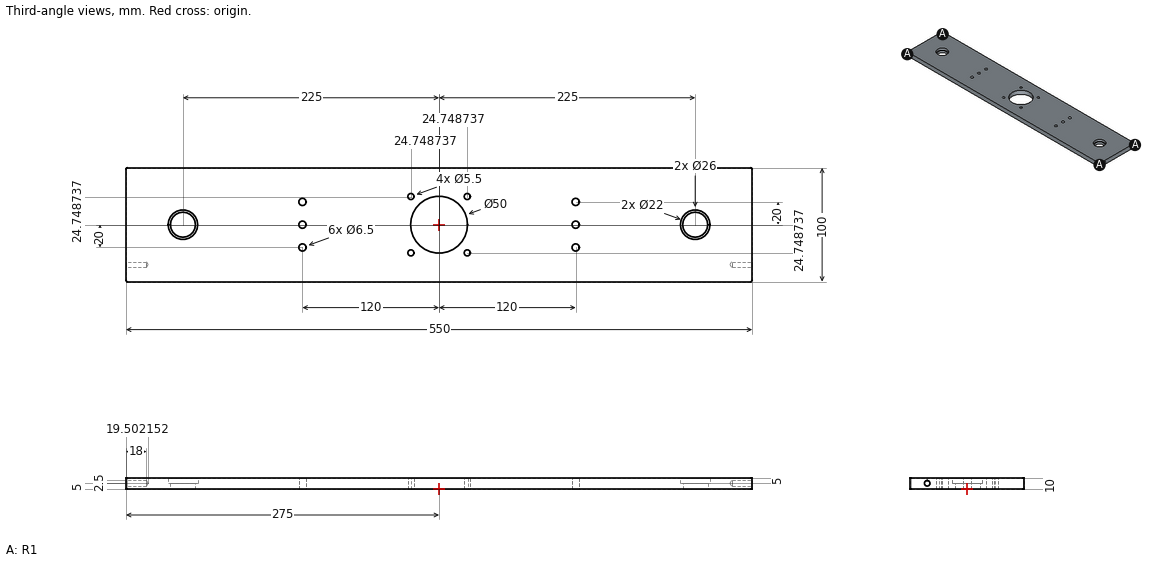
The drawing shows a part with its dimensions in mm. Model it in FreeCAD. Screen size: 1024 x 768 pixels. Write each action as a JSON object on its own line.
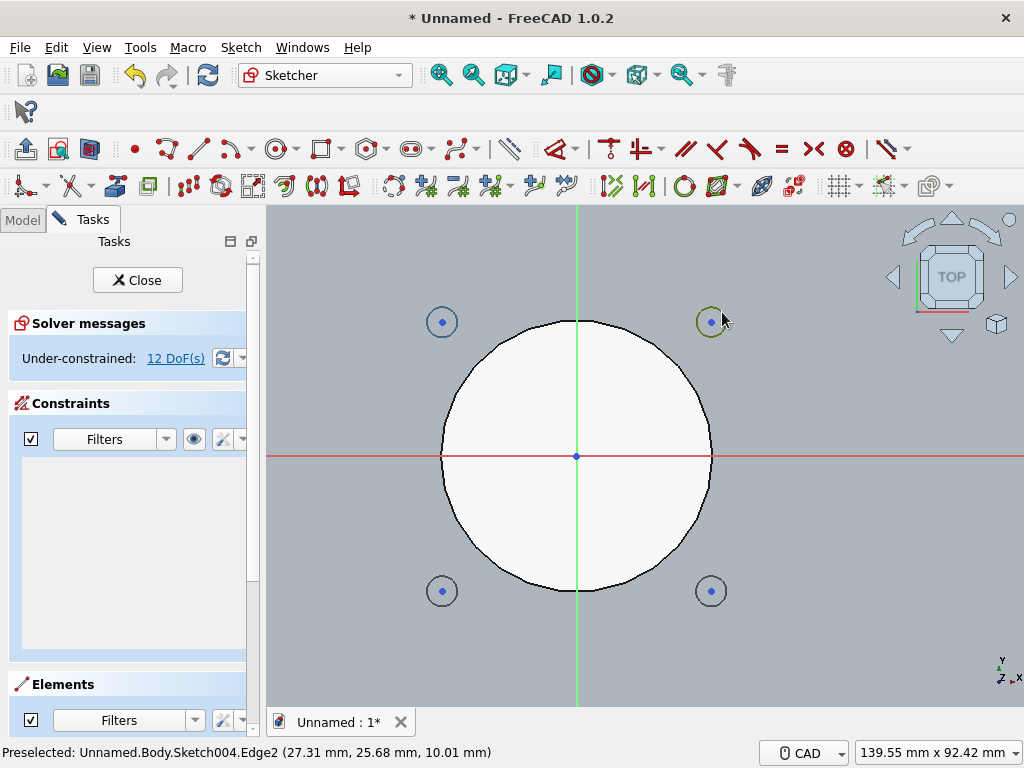
{"action": "left_click", "coordinate": [722, 581]}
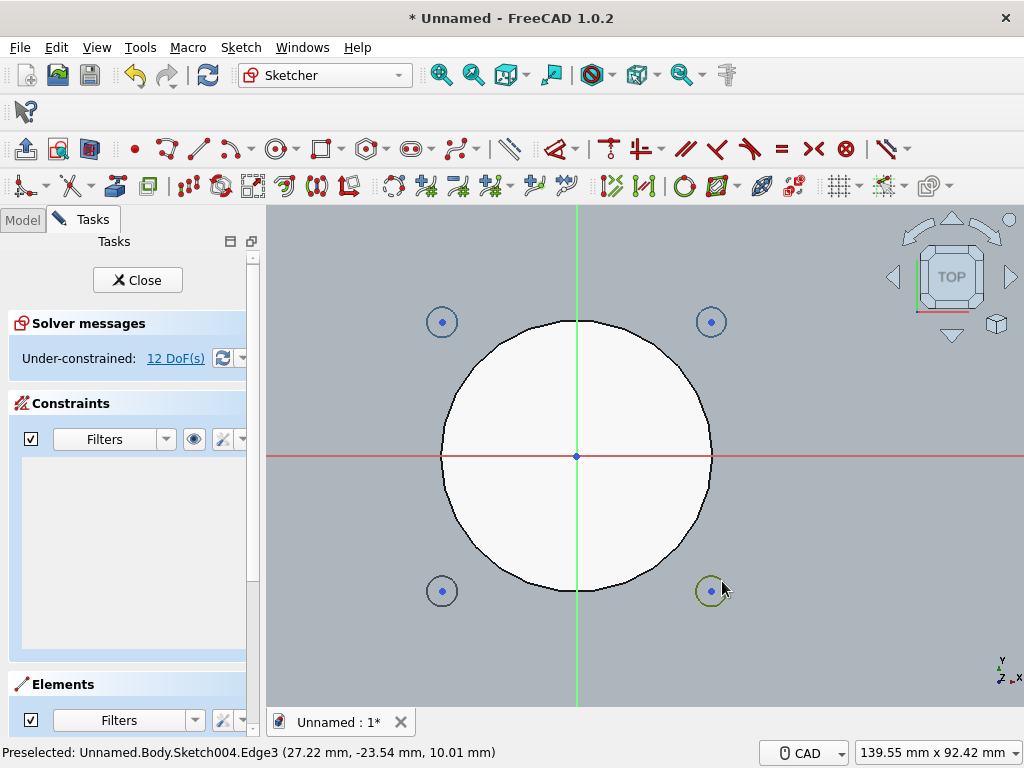
{"action": "left_click", "coordinate": [453, 581]}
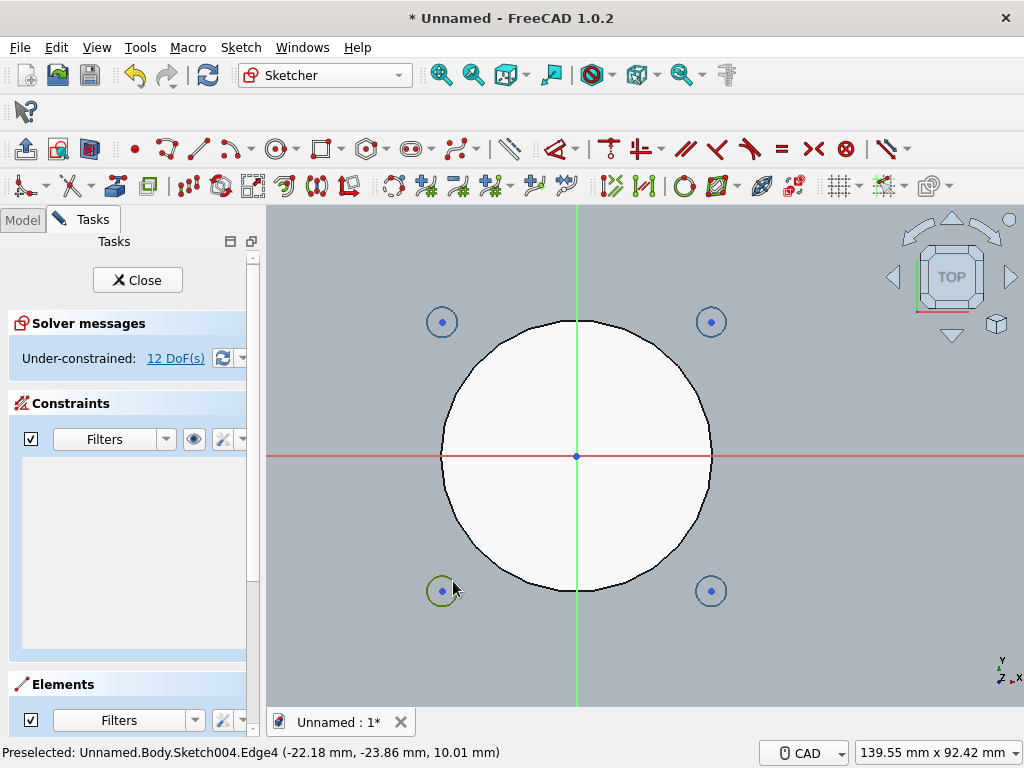
{"action": "key", "text": "e"}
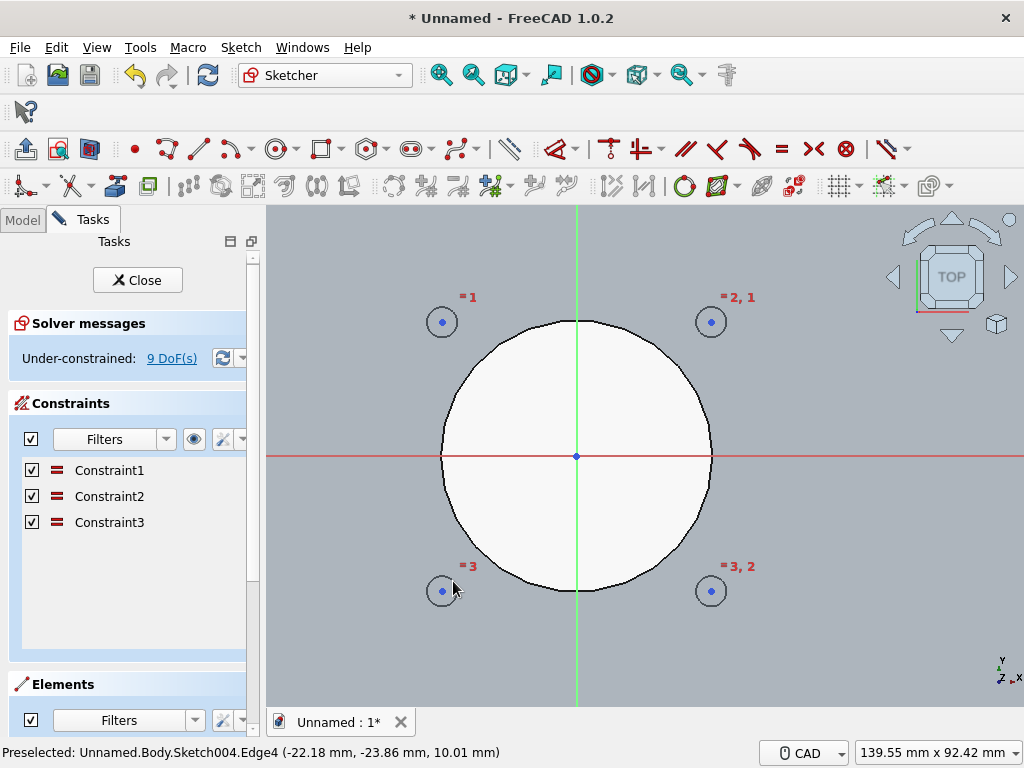
{"action": "left_click", "coordinate": [442, 322]}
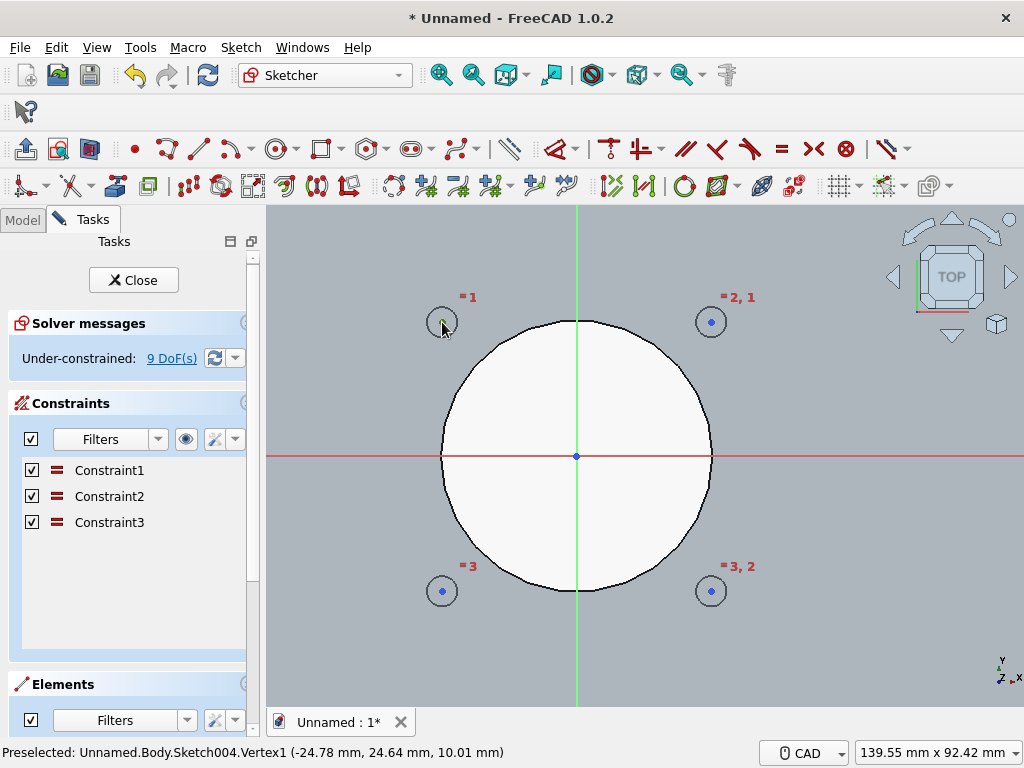
{"action": "left_click", "coordinate": [711, 322]}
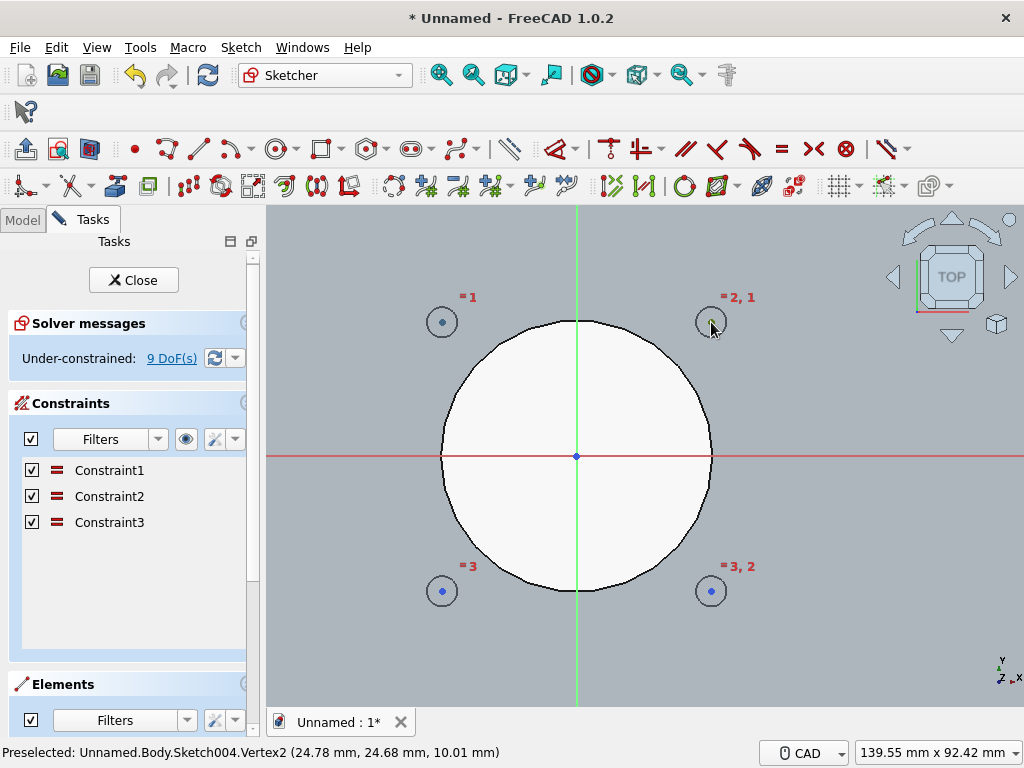
{"action": "key", "text": "h"}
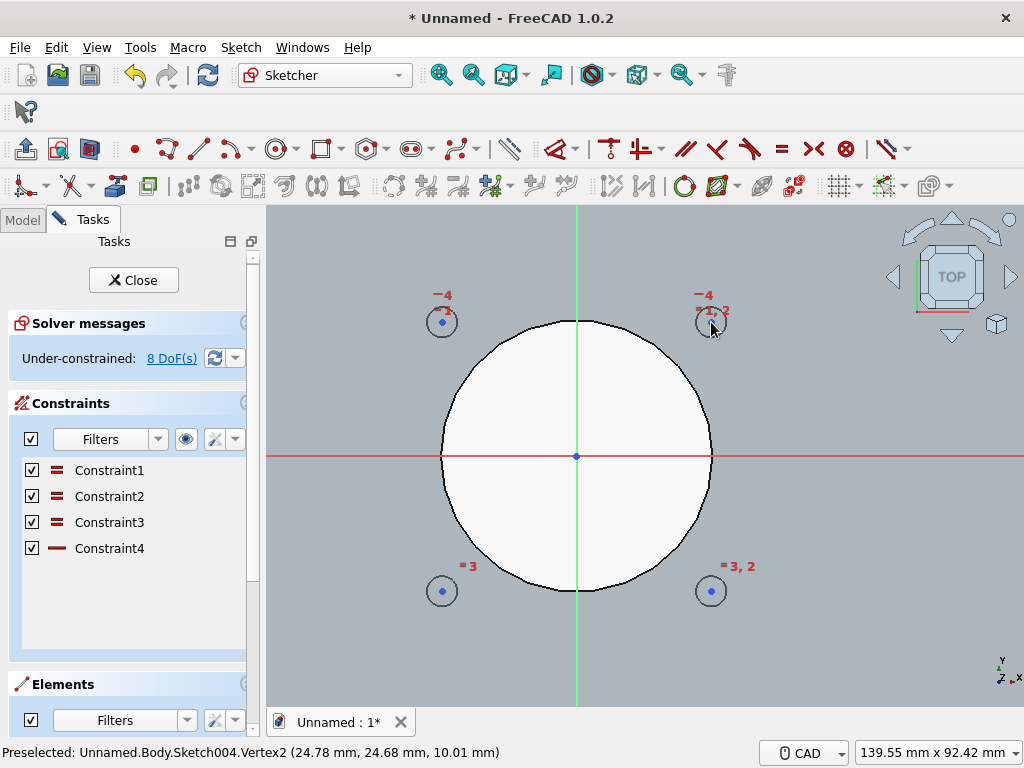
{"action": "left_click", "coordinate": [711, 322]}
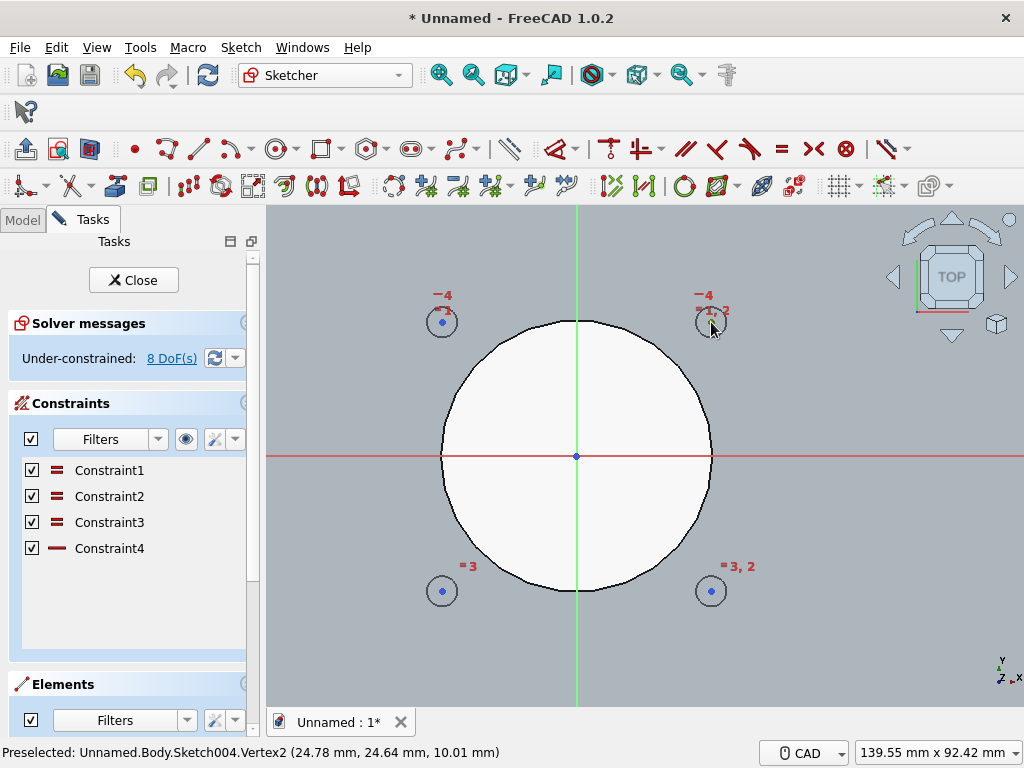
{"action": "left_click", "coordinate": [711, 591]}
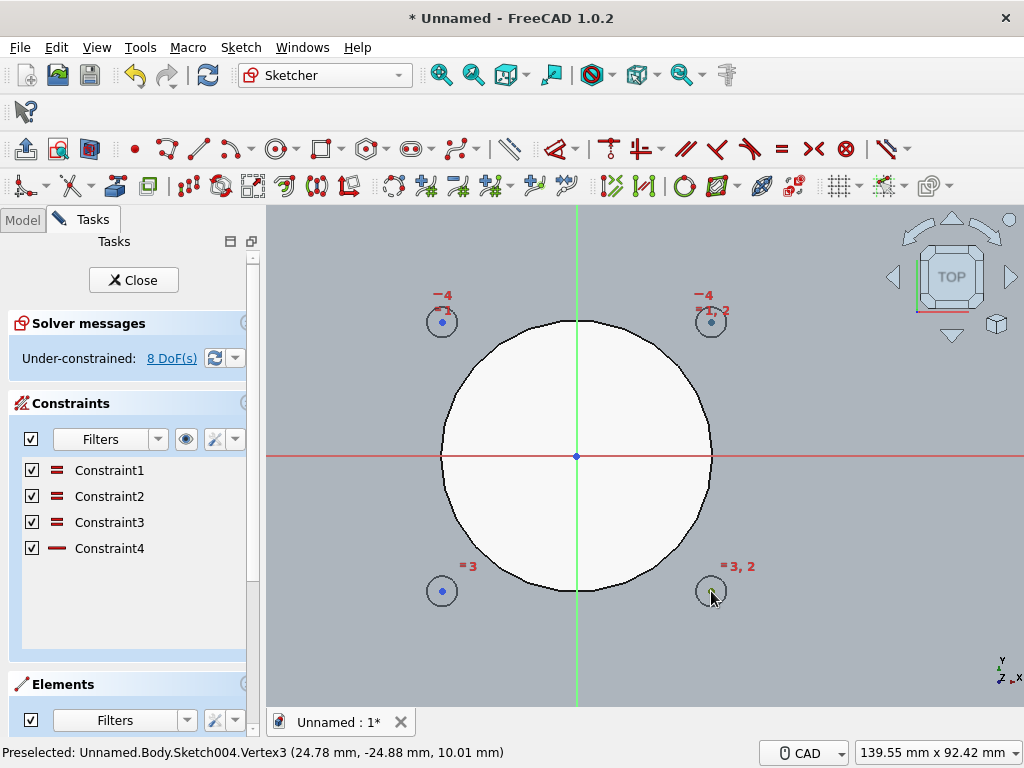
{"action": "key", "text": "v"}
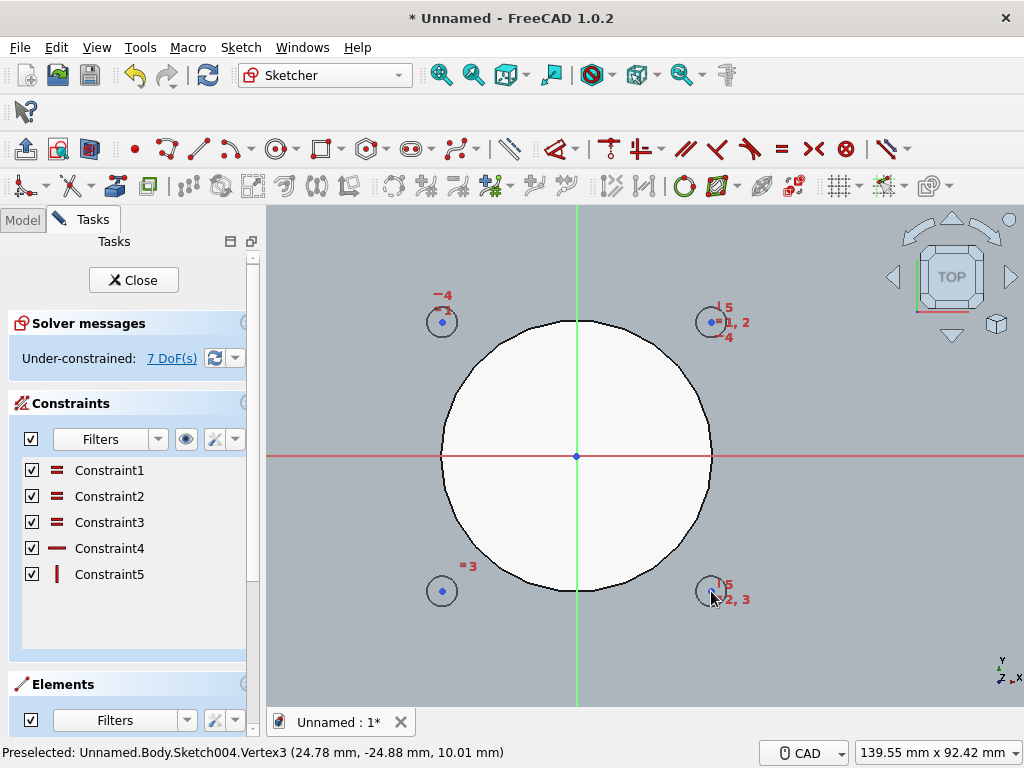
{"action": "left_click", "coordinate": [442, 322]}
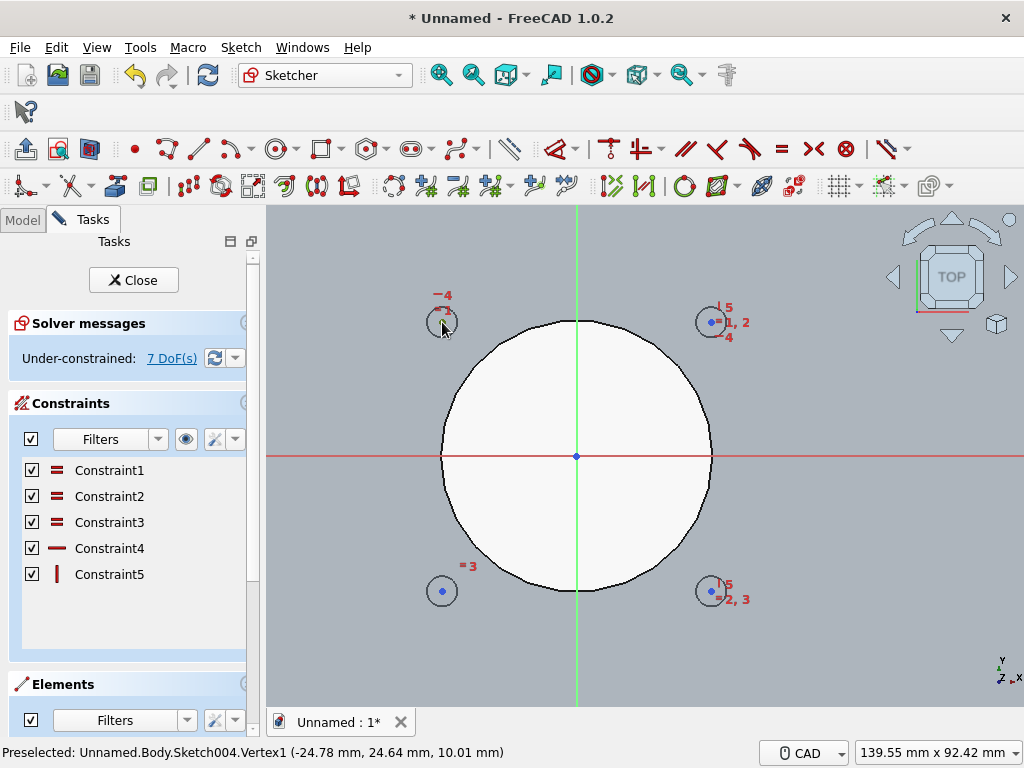
{"action": "left_click", "coordinate": [442, 591]}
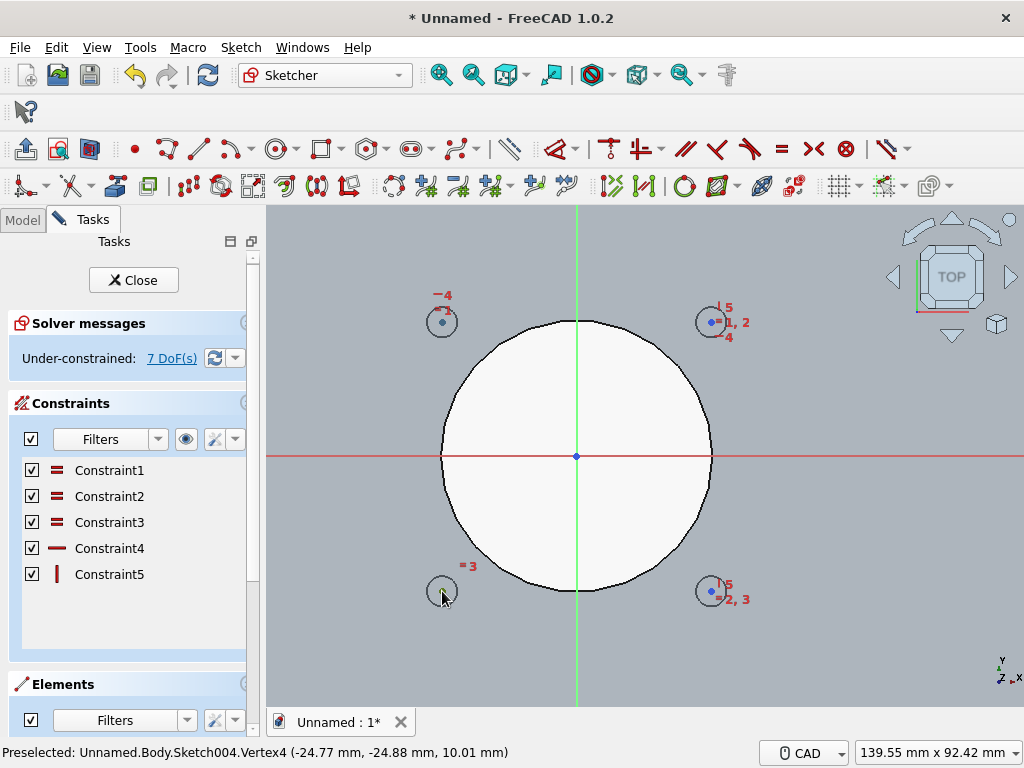
{"action": "key", "text": "v"}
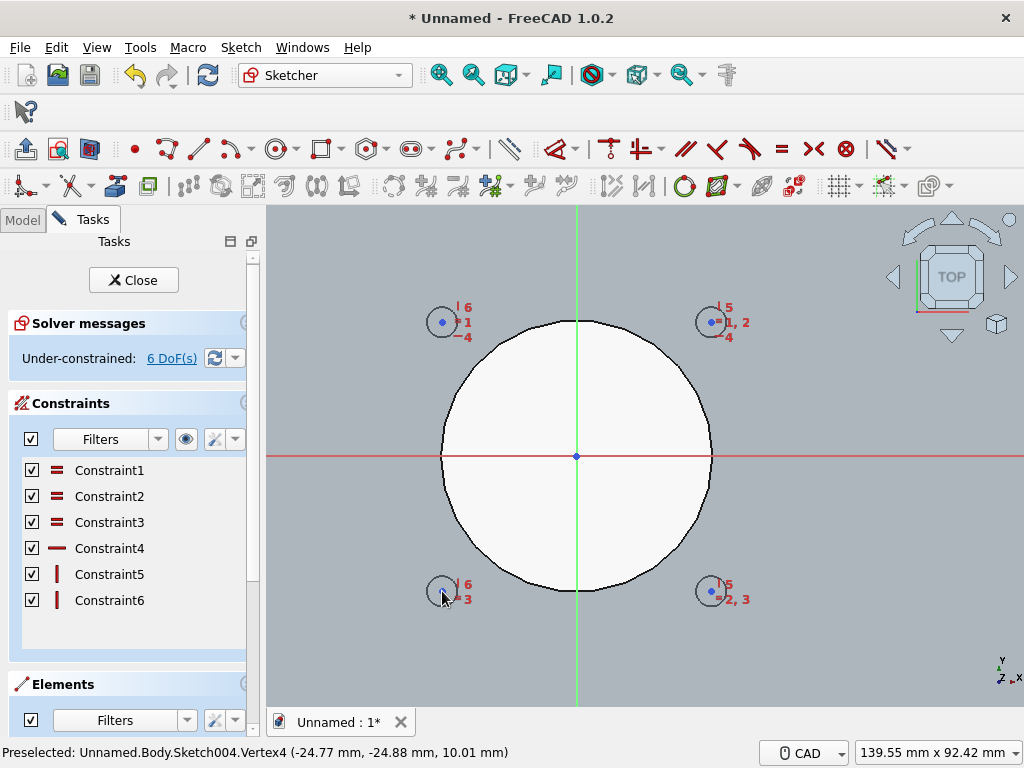
{"action": "left_click", "coordinate": [711, 591]}